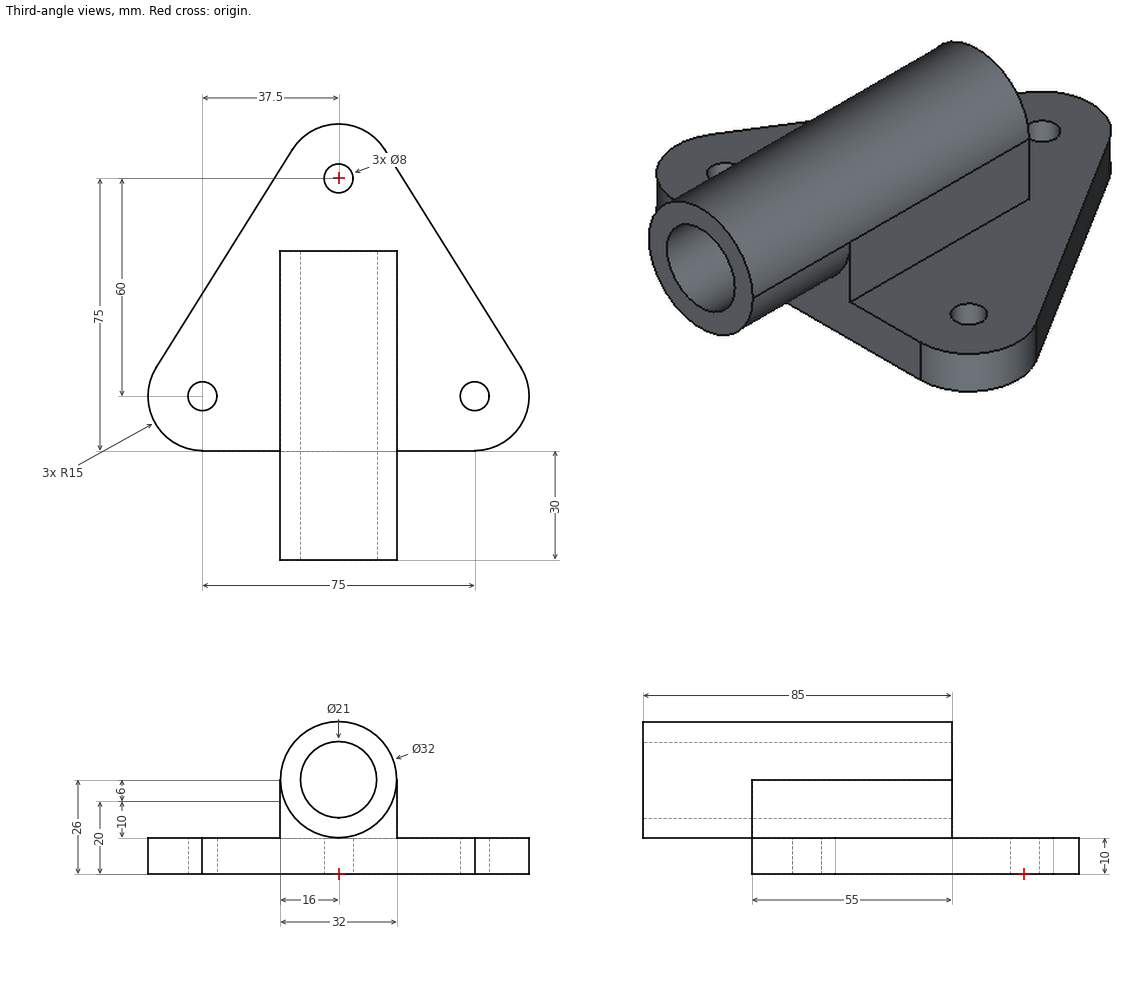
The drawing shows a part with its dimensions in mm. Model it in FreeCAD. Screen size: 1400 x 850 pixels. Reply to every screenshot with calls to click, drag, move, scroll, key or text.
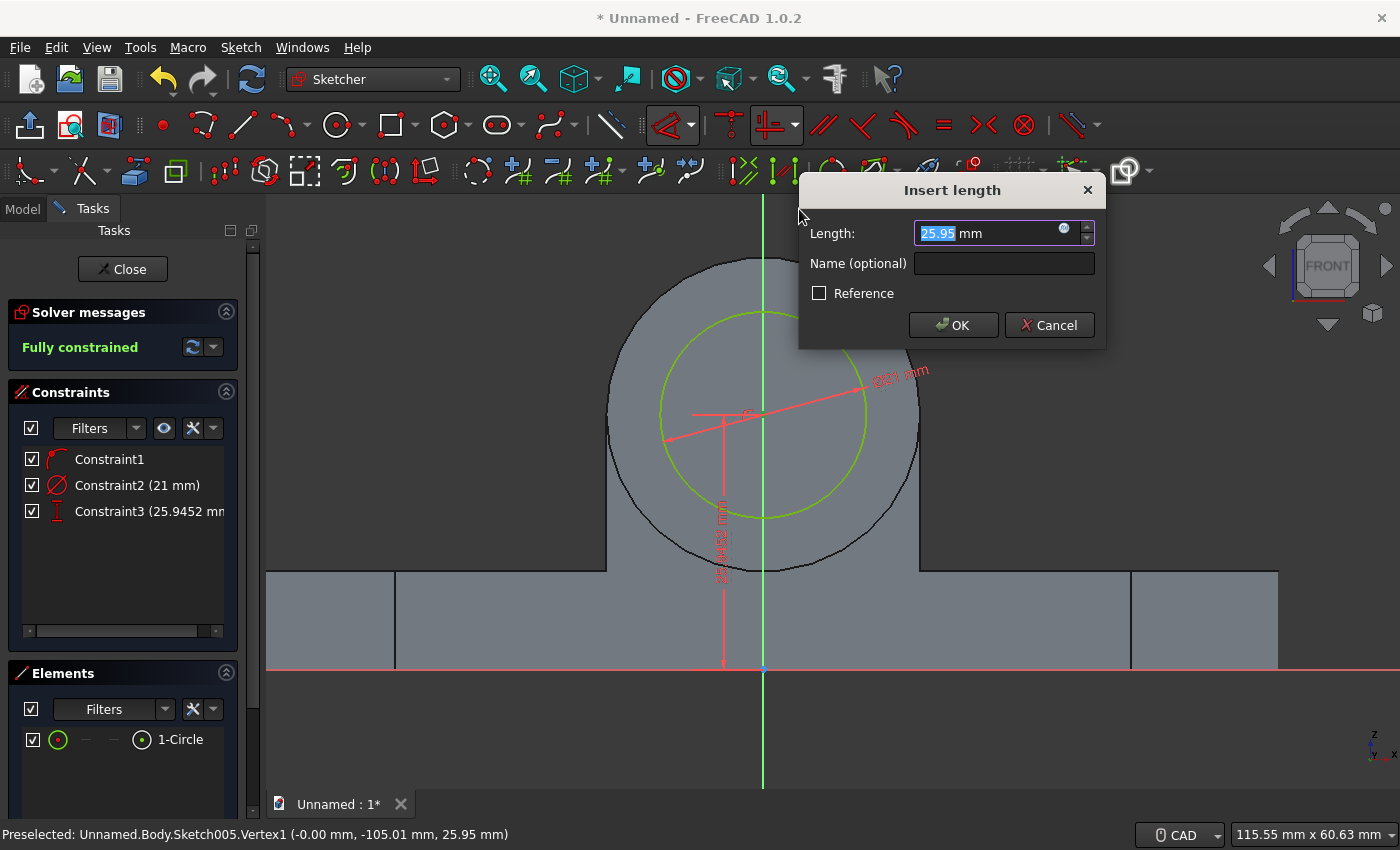
text(26)
key(Return)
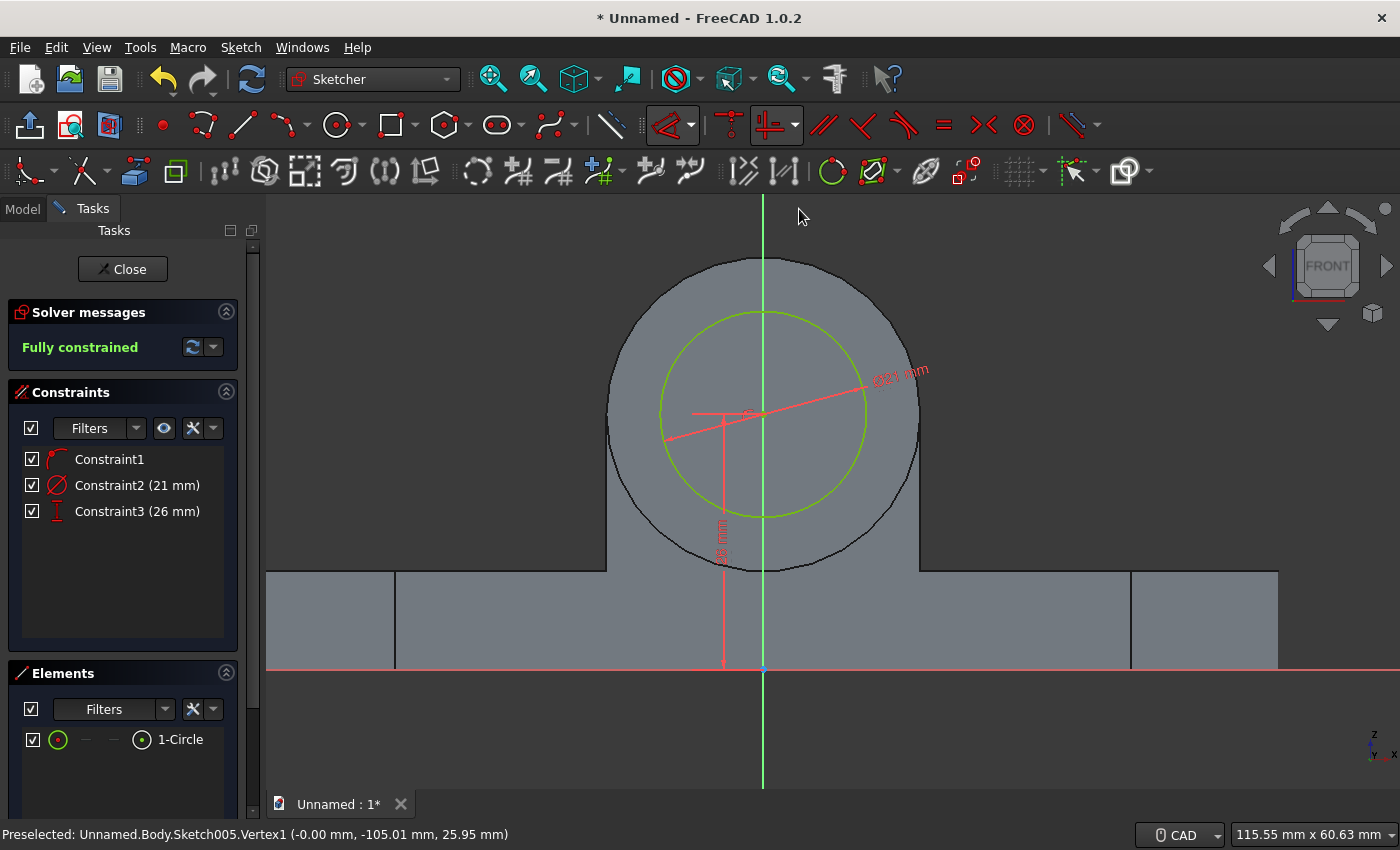
click(123, 269)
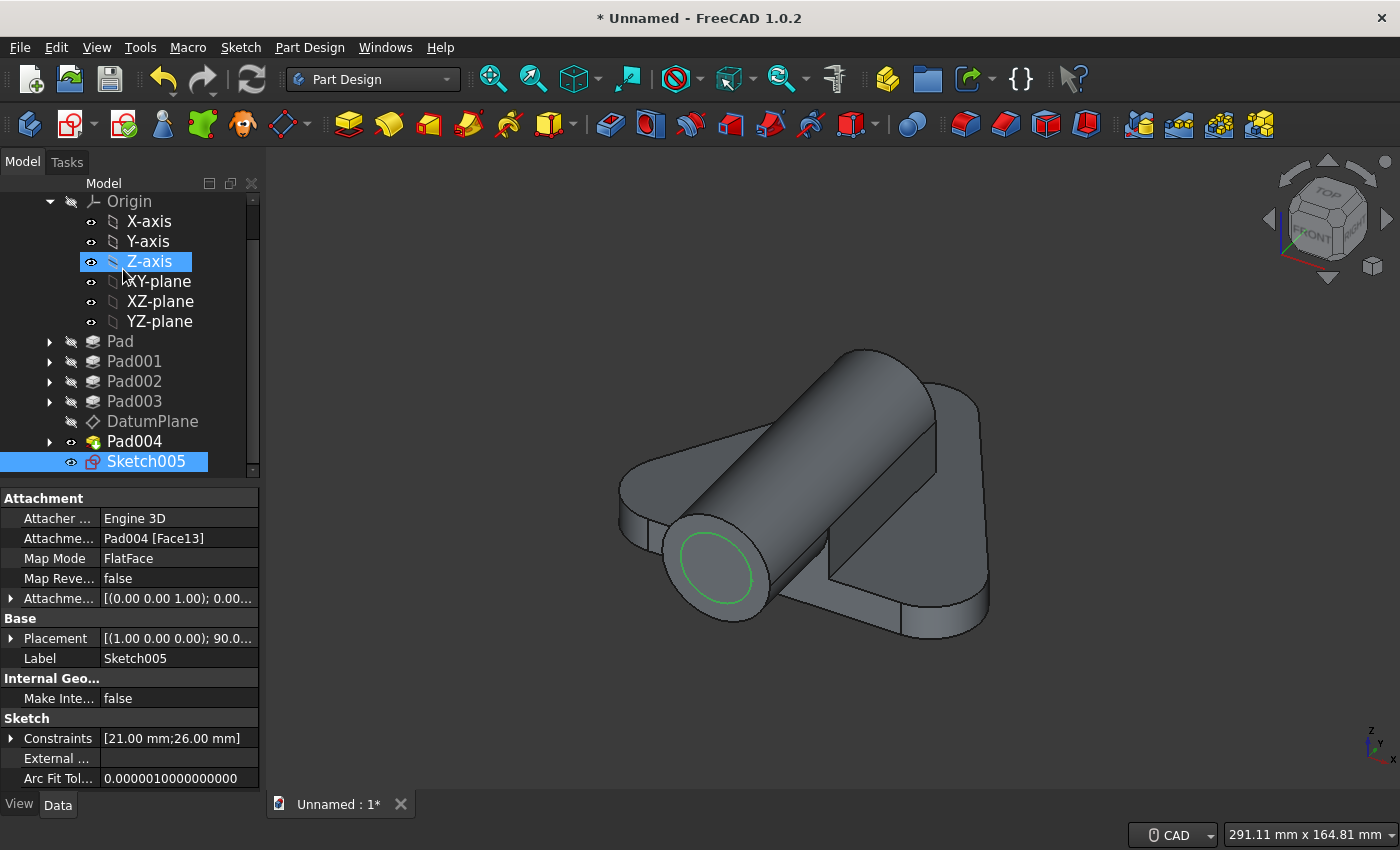
click(612, 124)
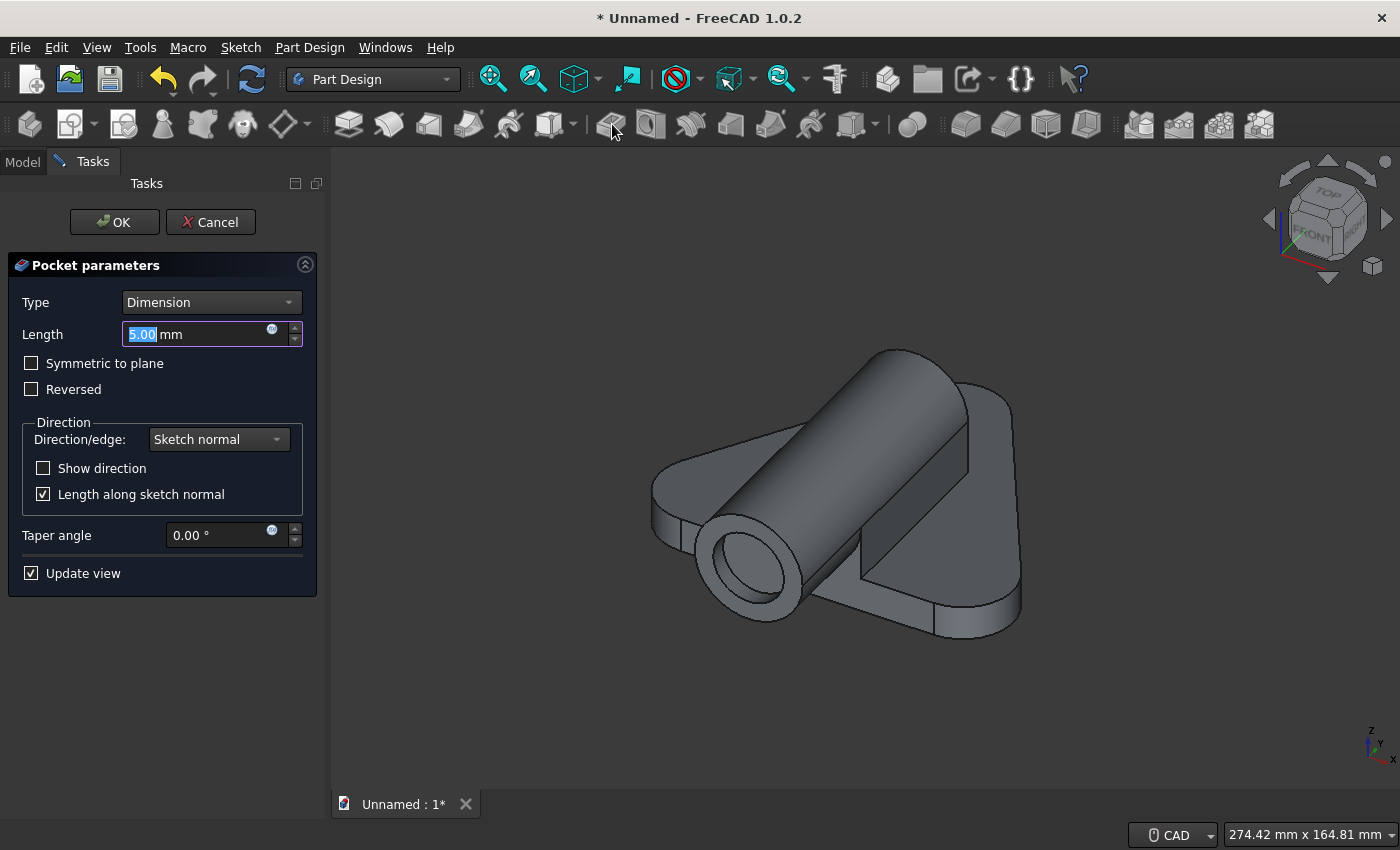
text(85)
key(Tab)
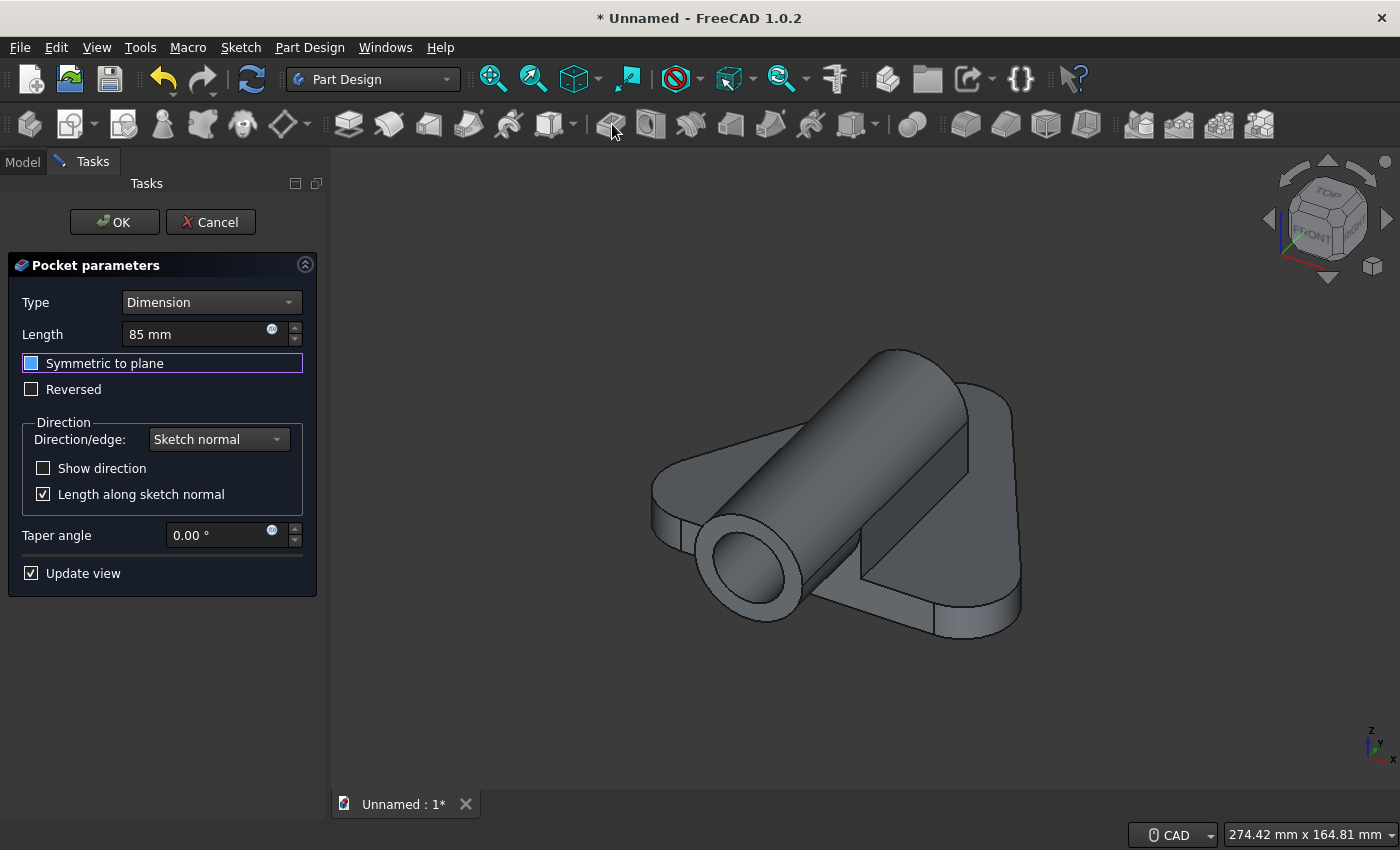
click(115, 222)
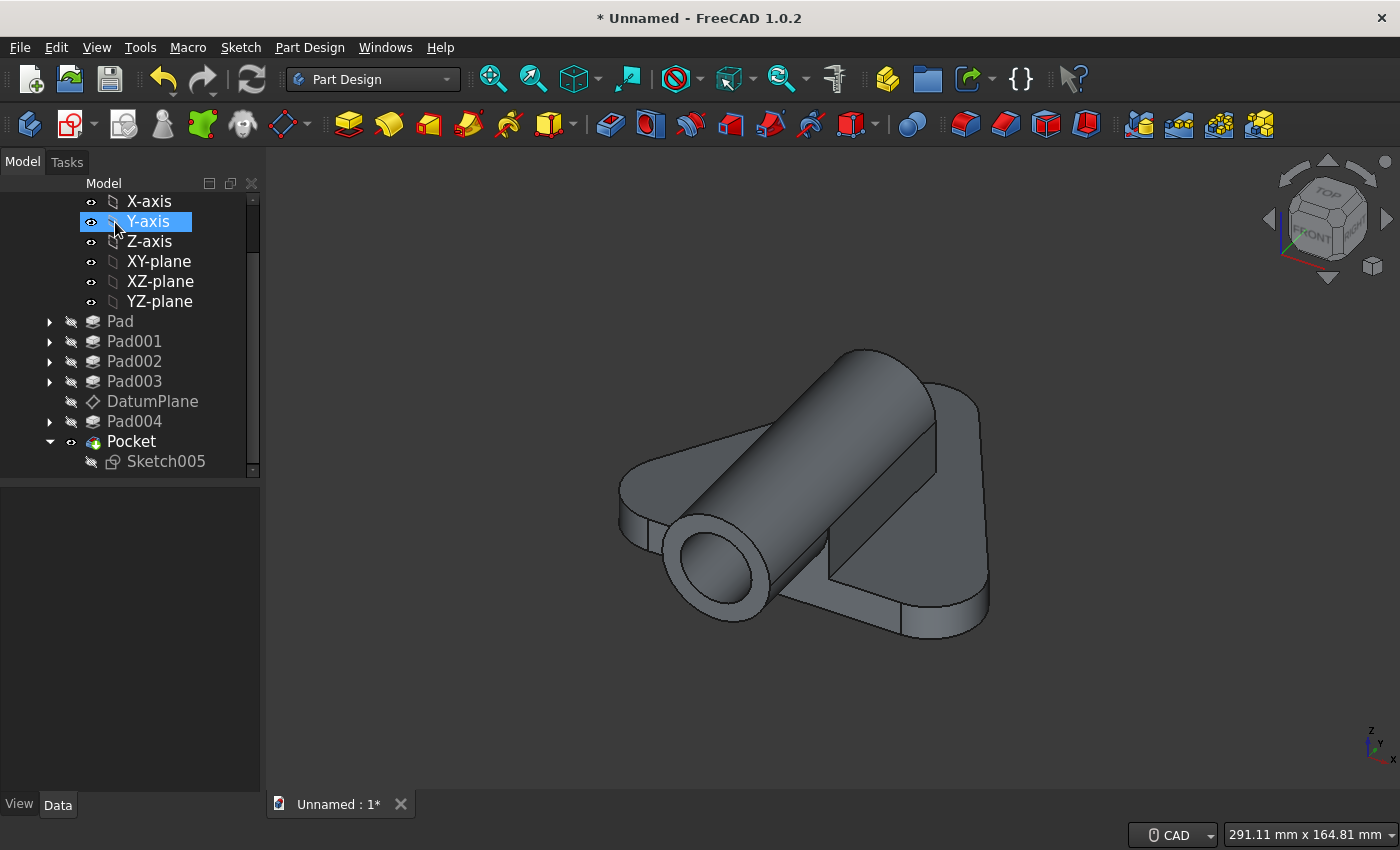
click(913, 556)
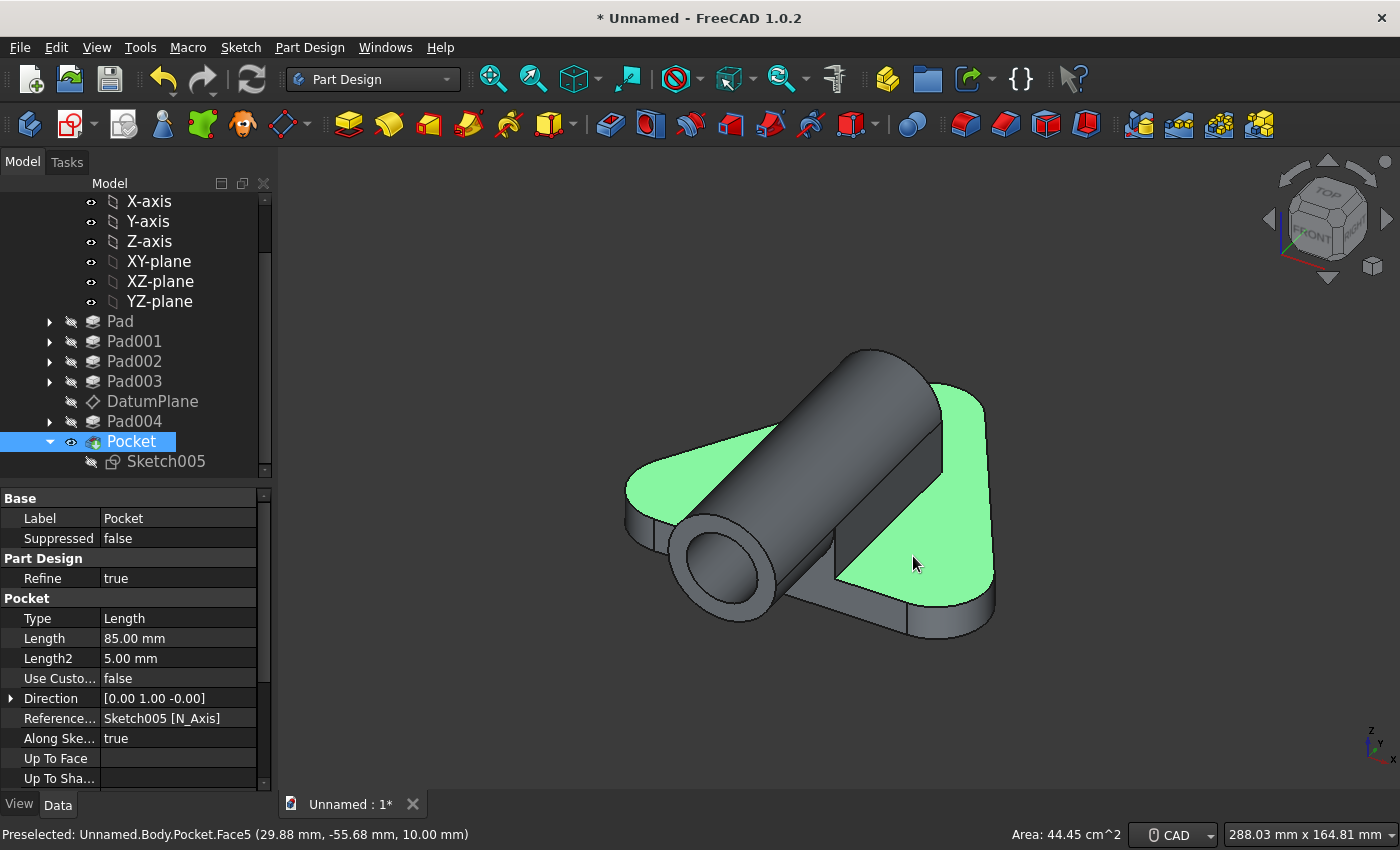
click(70, 124)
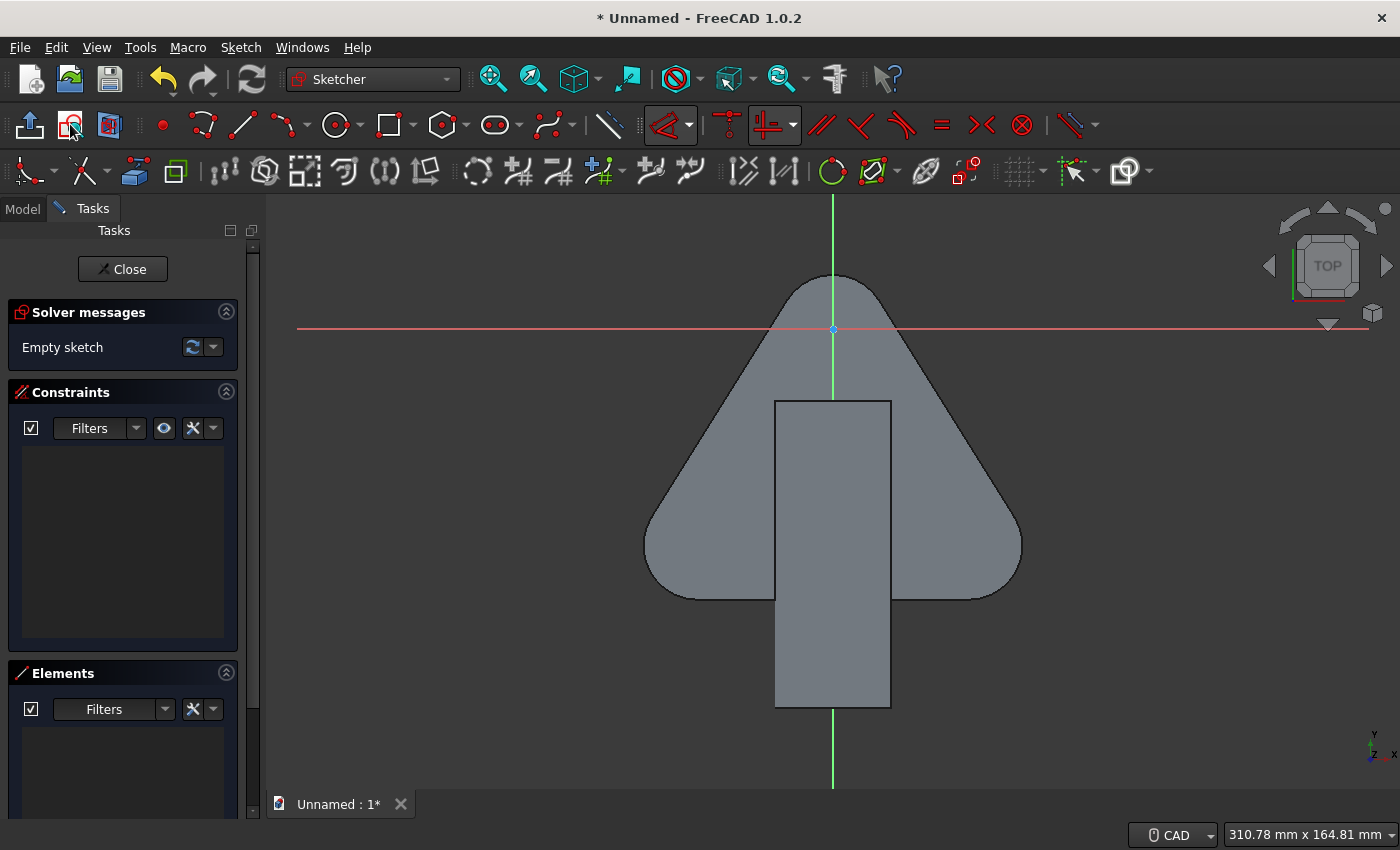
click(110, 126)